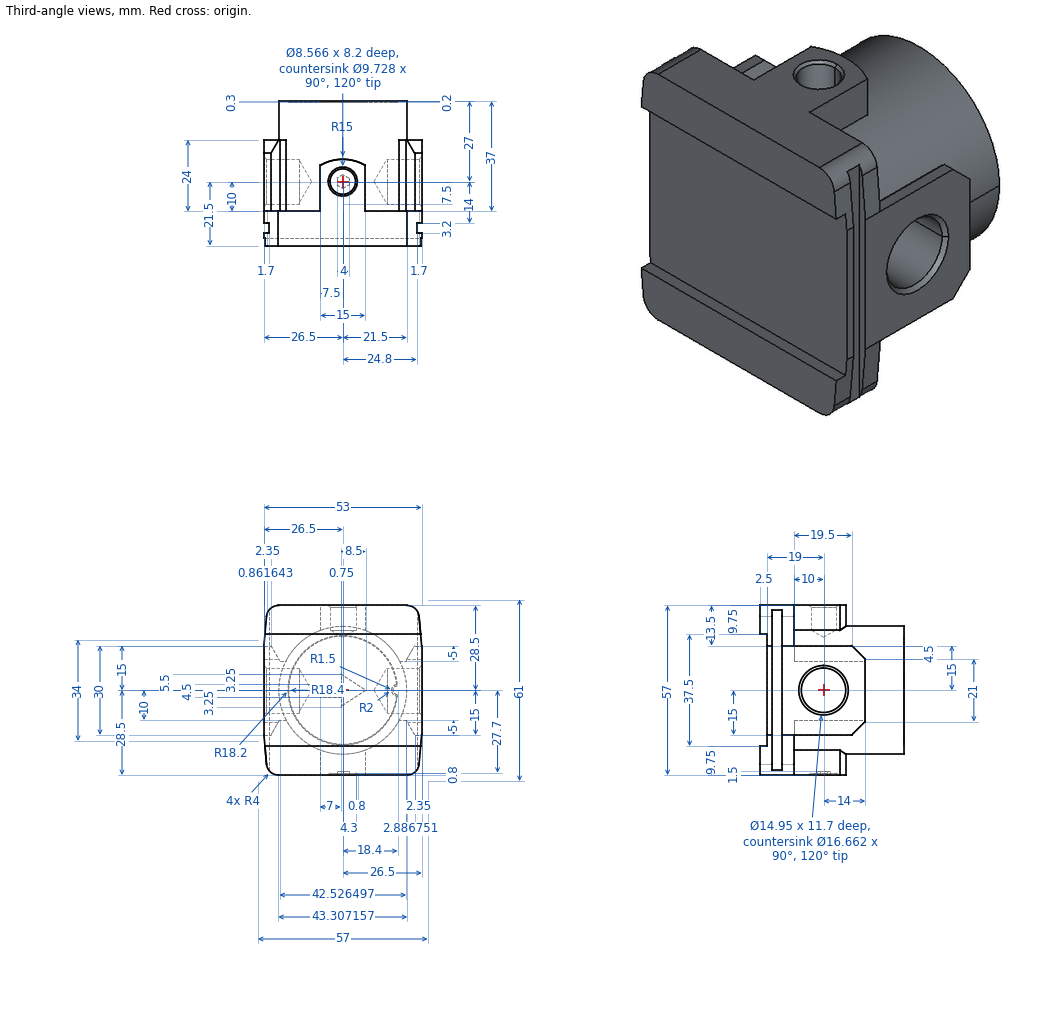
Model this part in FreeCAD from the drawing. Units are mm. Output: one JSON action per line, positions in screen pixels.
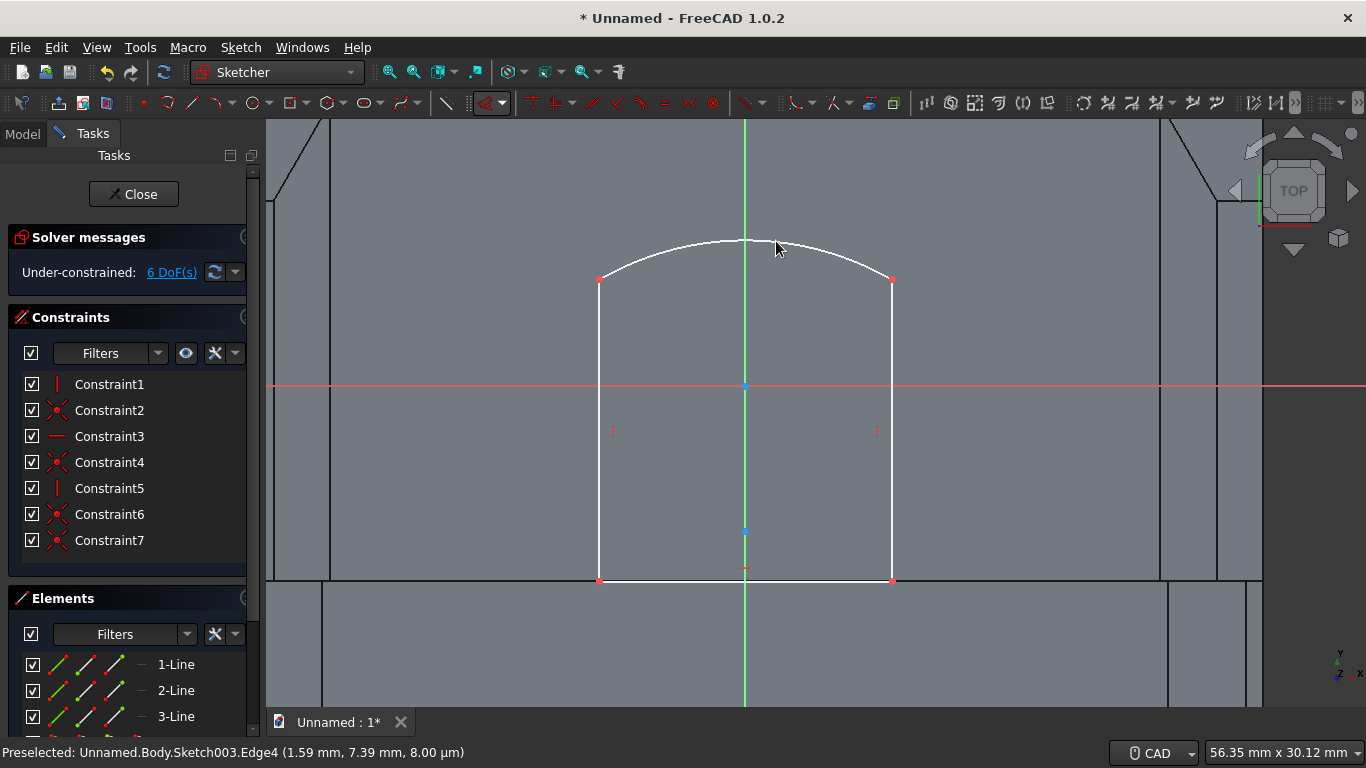
{"action": "left_click", "coordinate": [746, 531]}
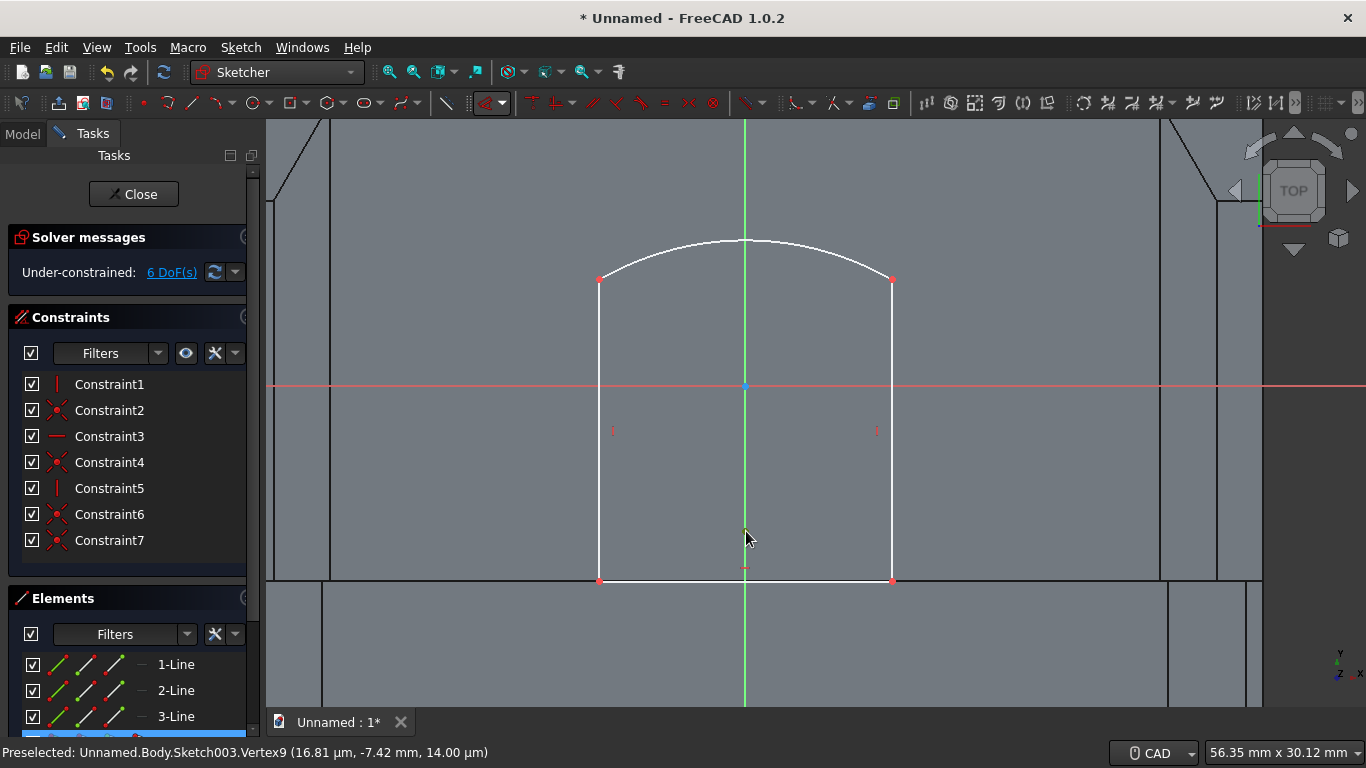
{"action": "left_click", "coordinate": [745, 641]}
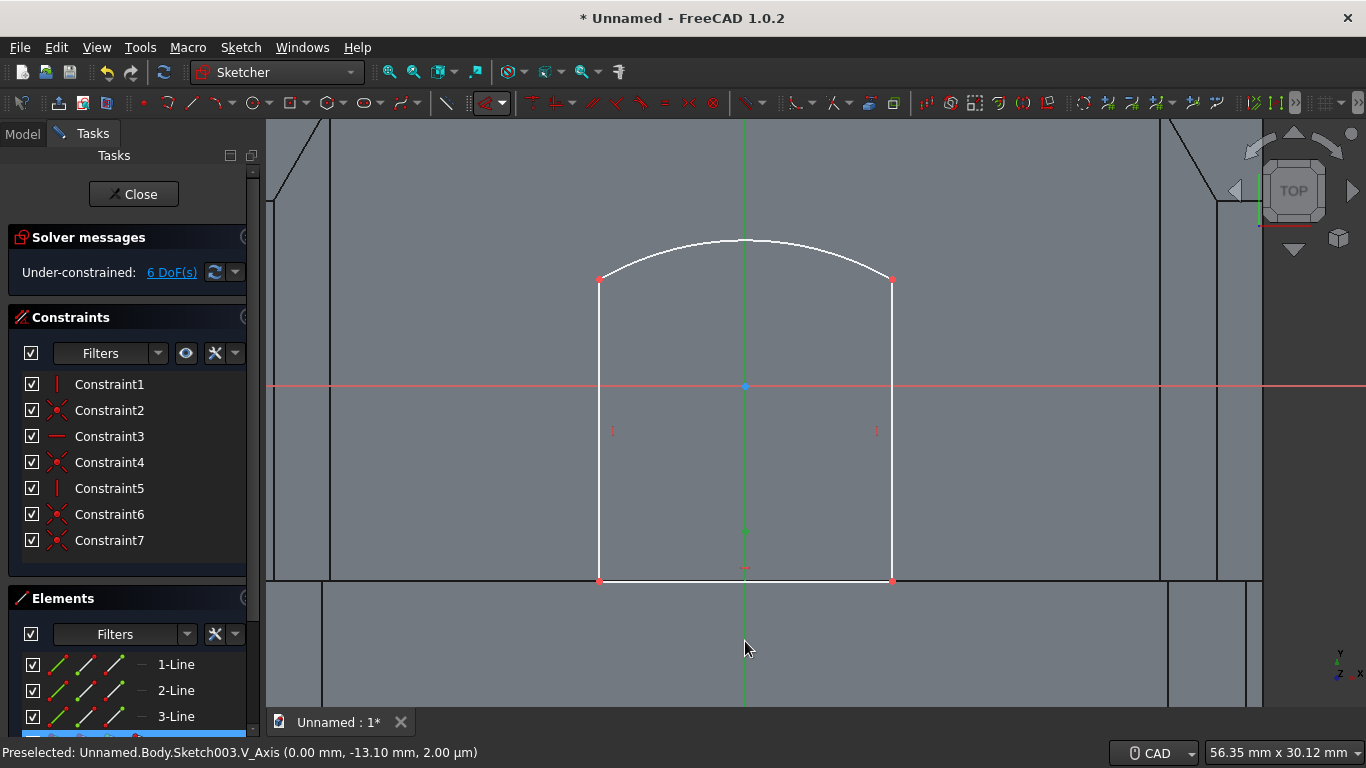
{"action": "left_click", "coordinate": [532, 104]}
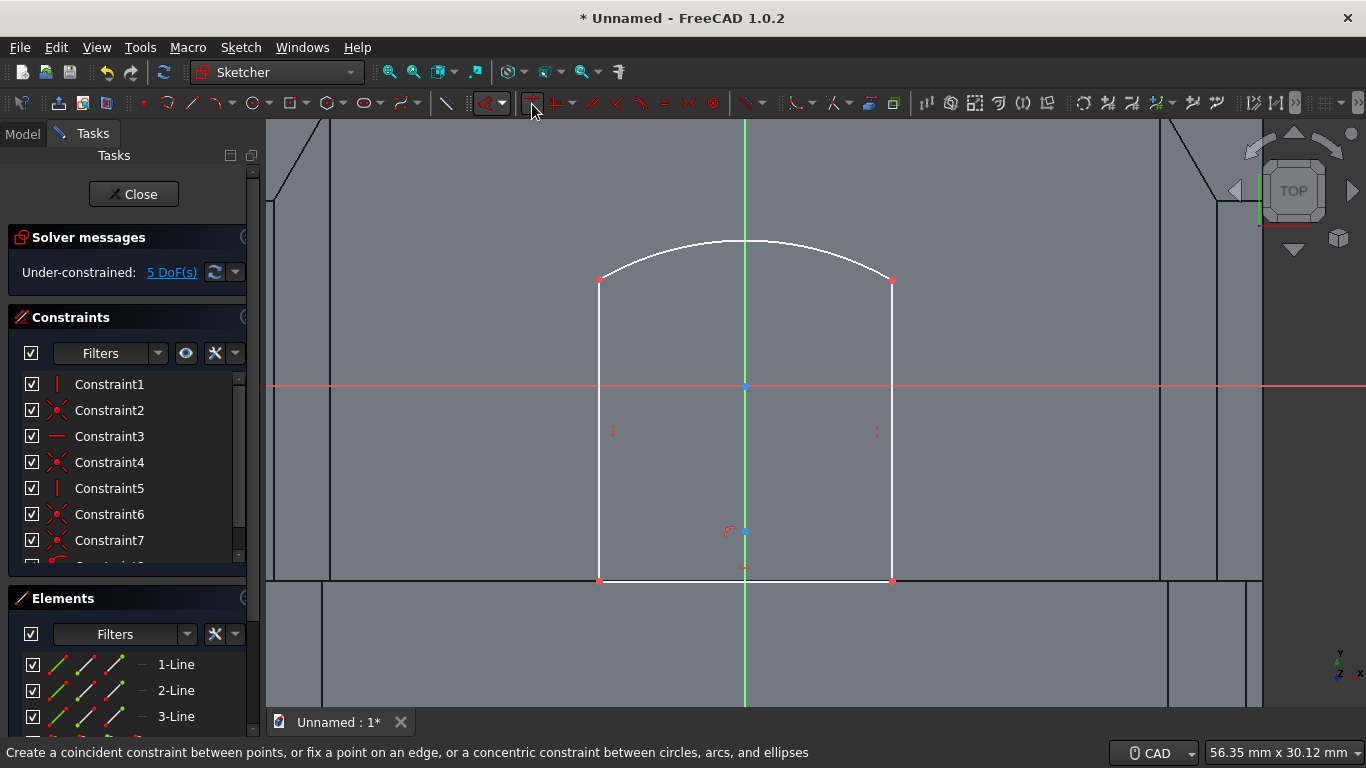
{"action": "left_click", "coordinate": [807, 247]}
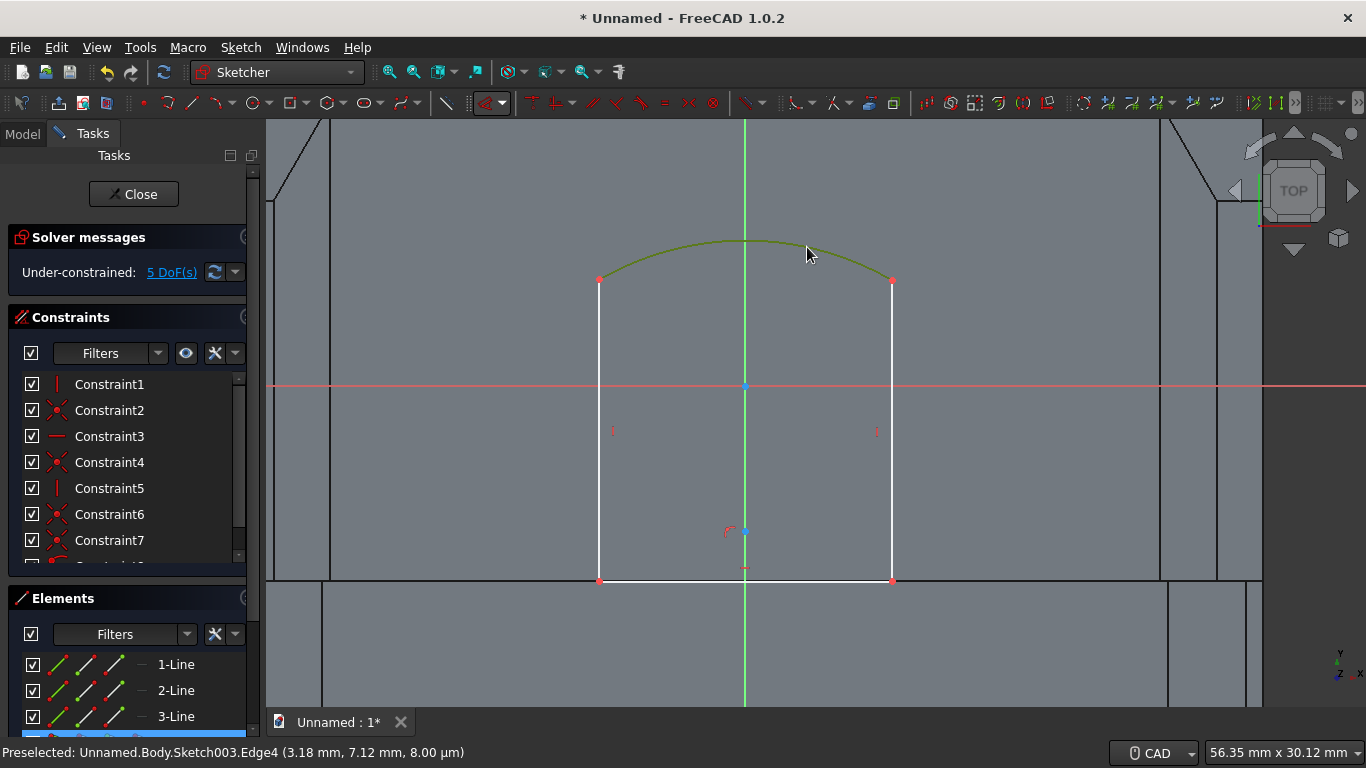
{"action": "left_click", "coordinate": [504, 104]}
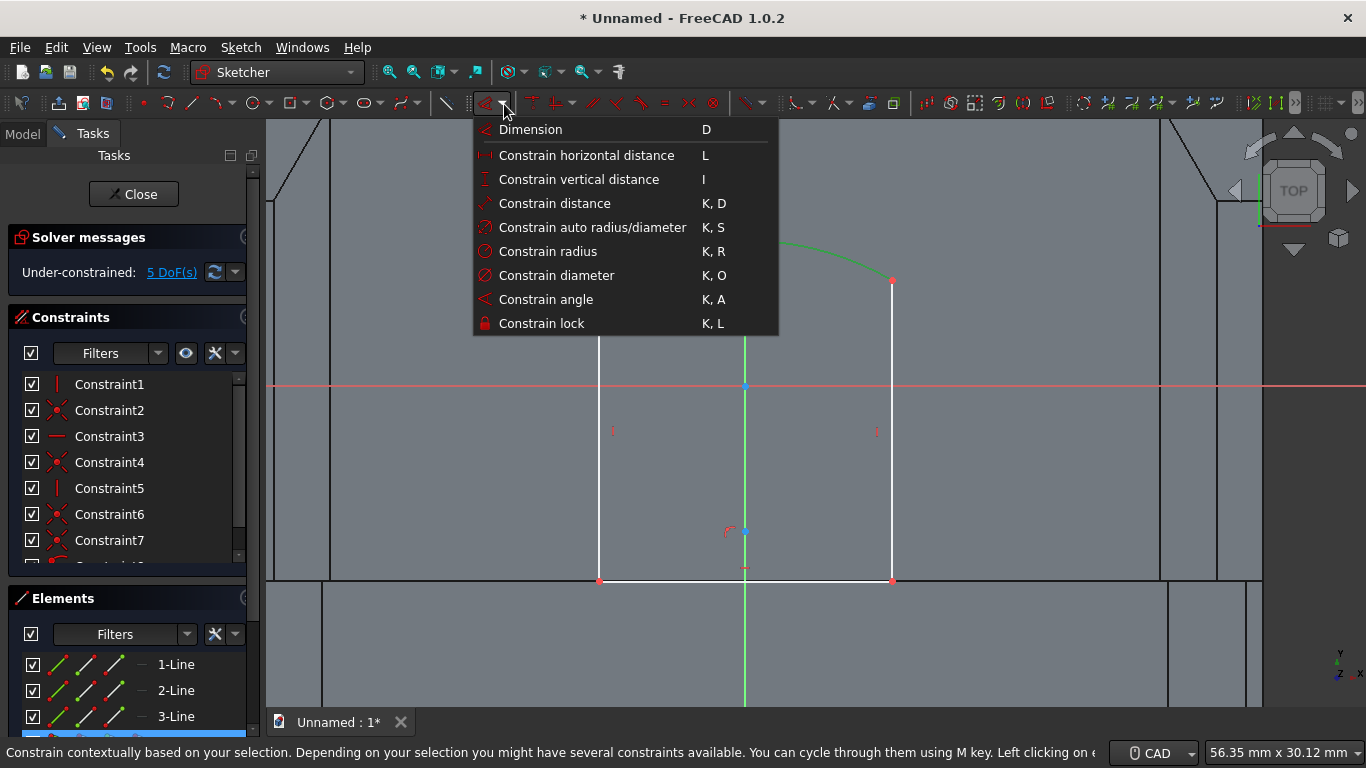
{"action": "left_click", "coordinate": [626, 251]}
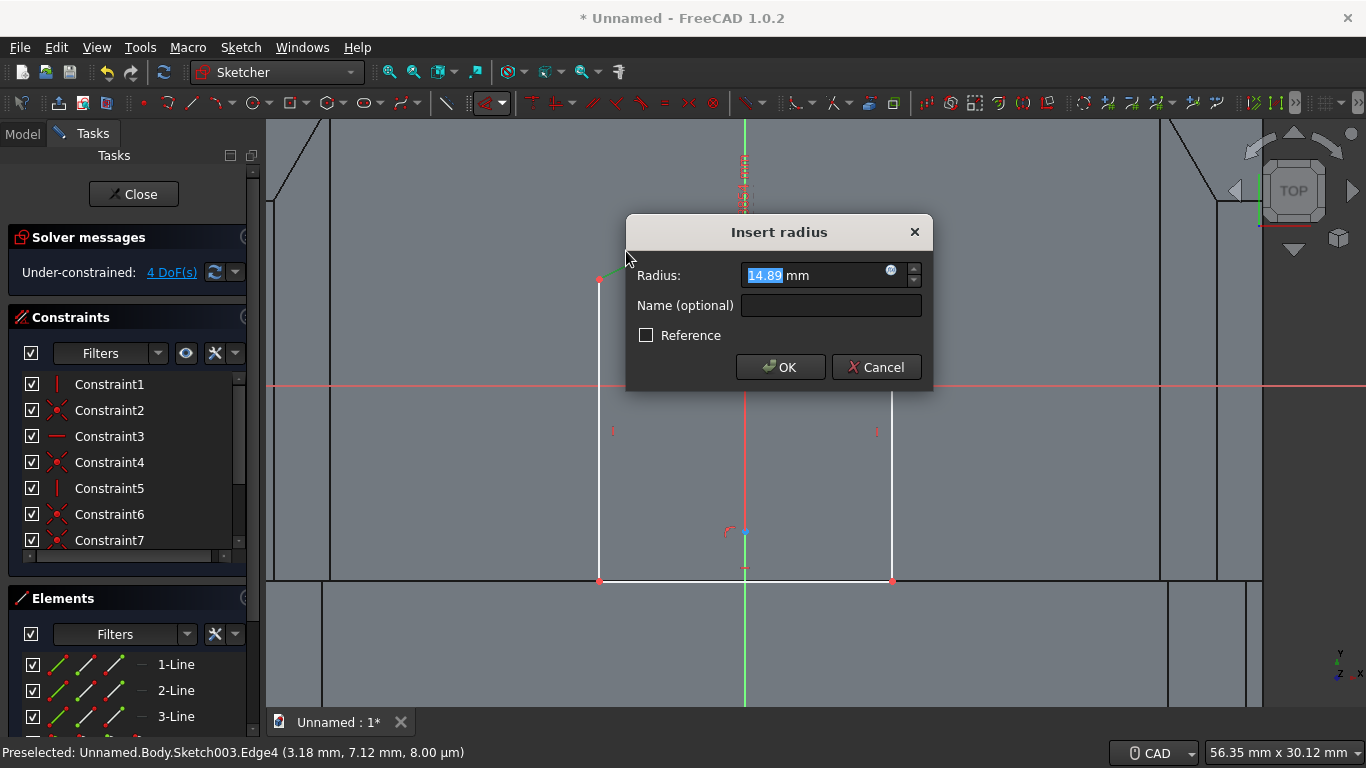
{"action": "type", "text": "15"}
{"action": "key", "text": "Return"}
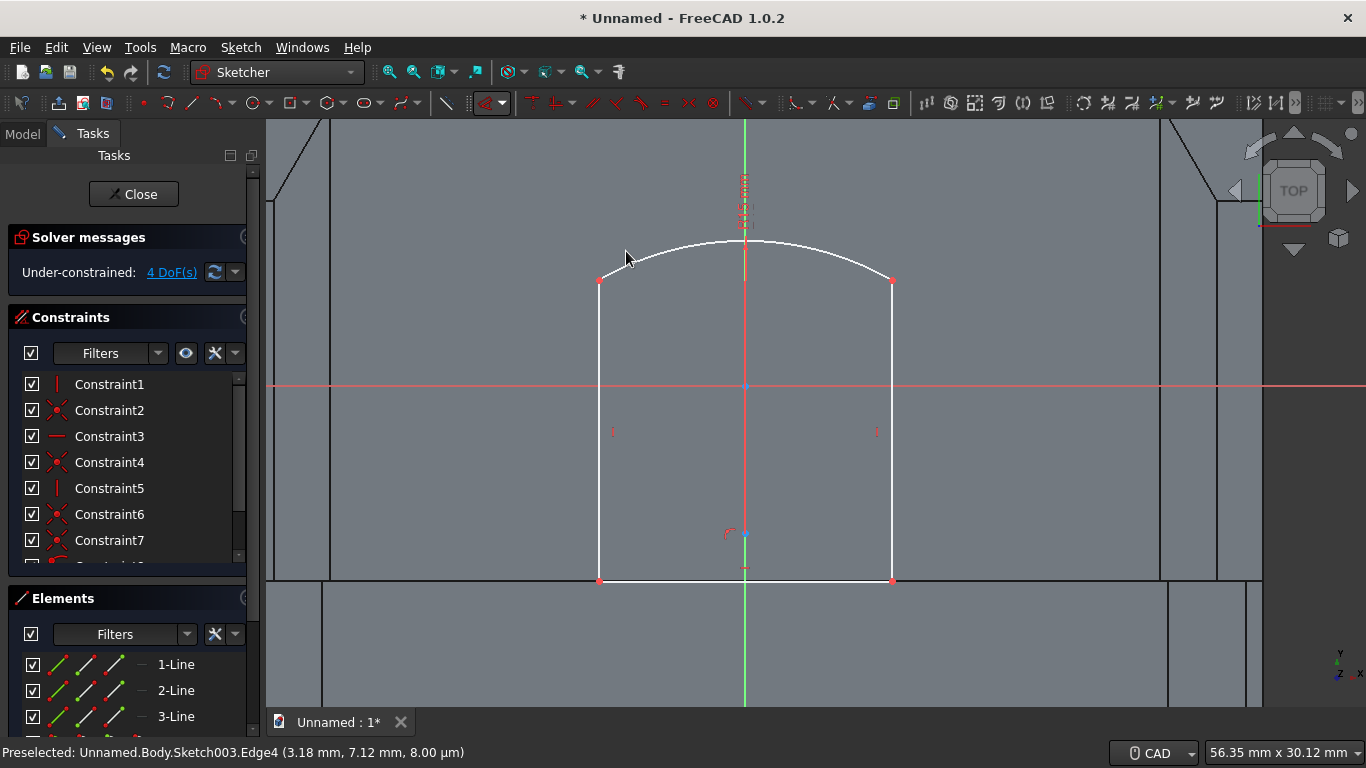
{"action": "left_click", "coordinate": [687, 582]}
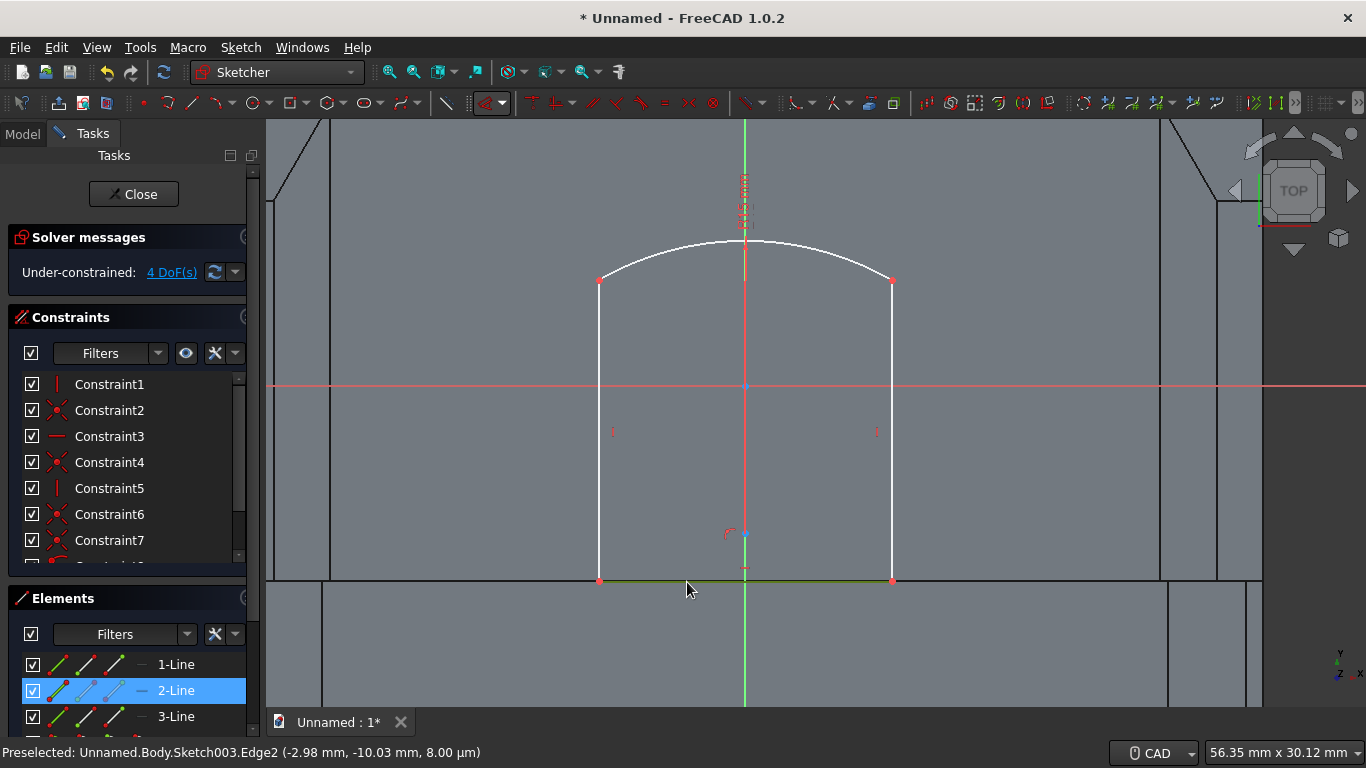
{"action": "left_click", "coordinate": [504, 104]}